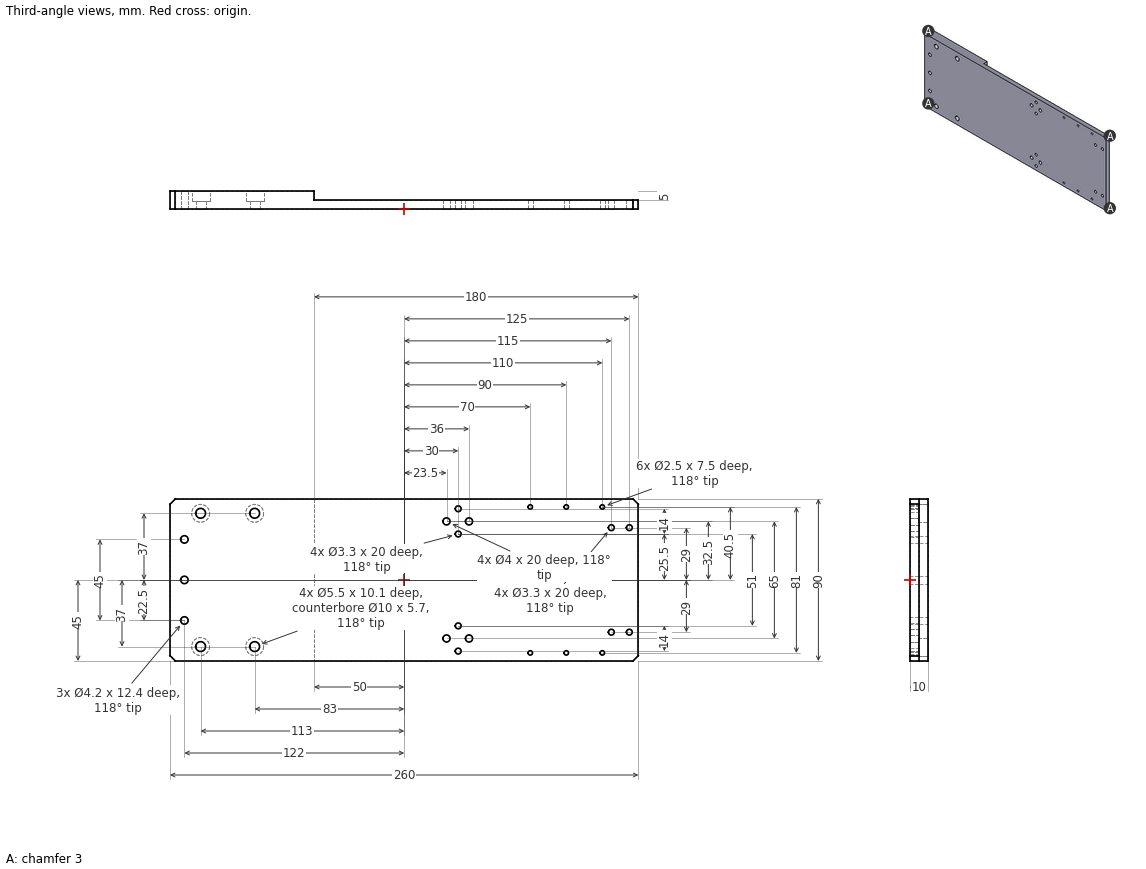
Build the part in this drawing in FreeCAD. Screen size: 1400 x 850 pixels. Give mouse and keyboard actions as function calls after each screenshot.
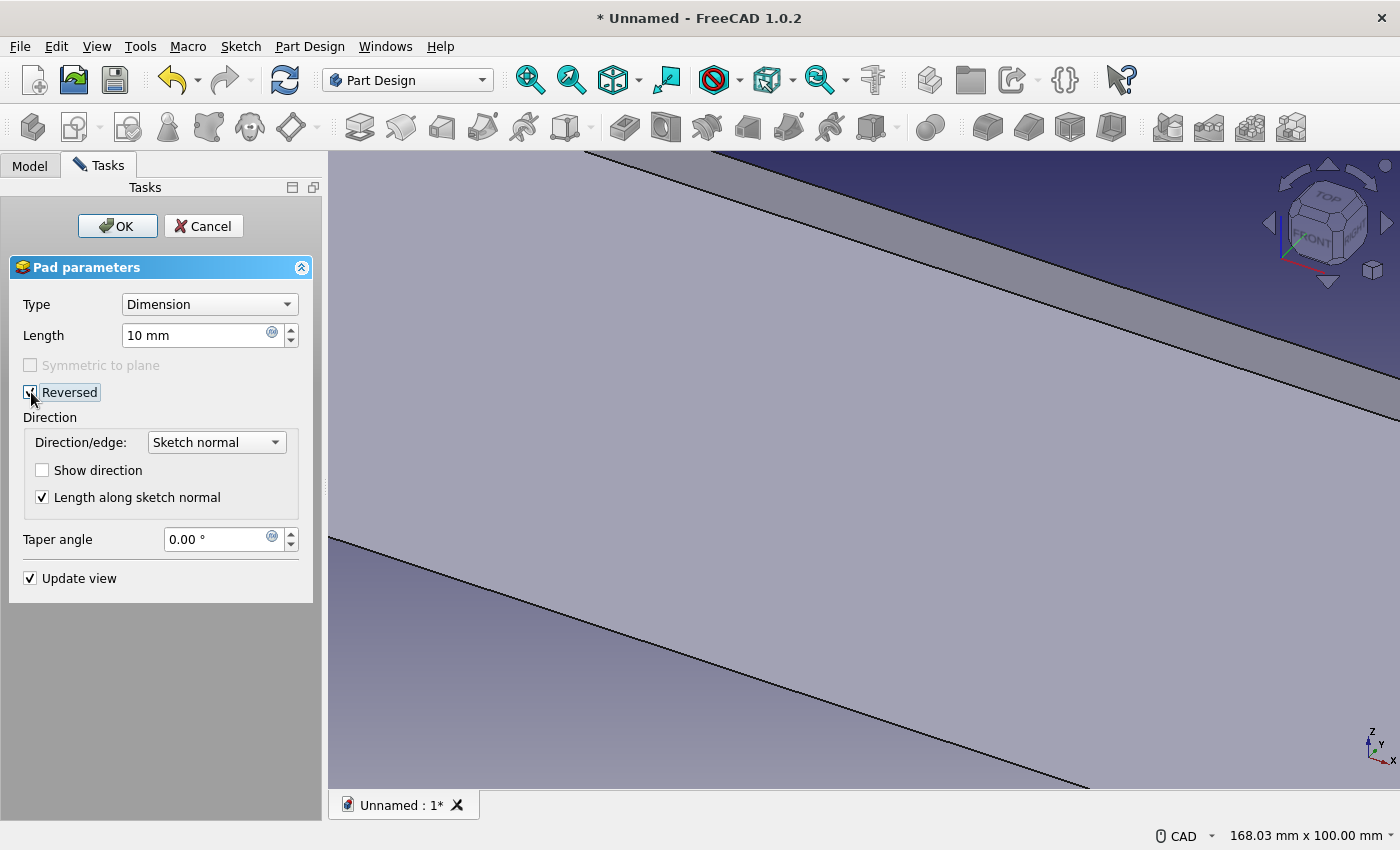
click(118, 226)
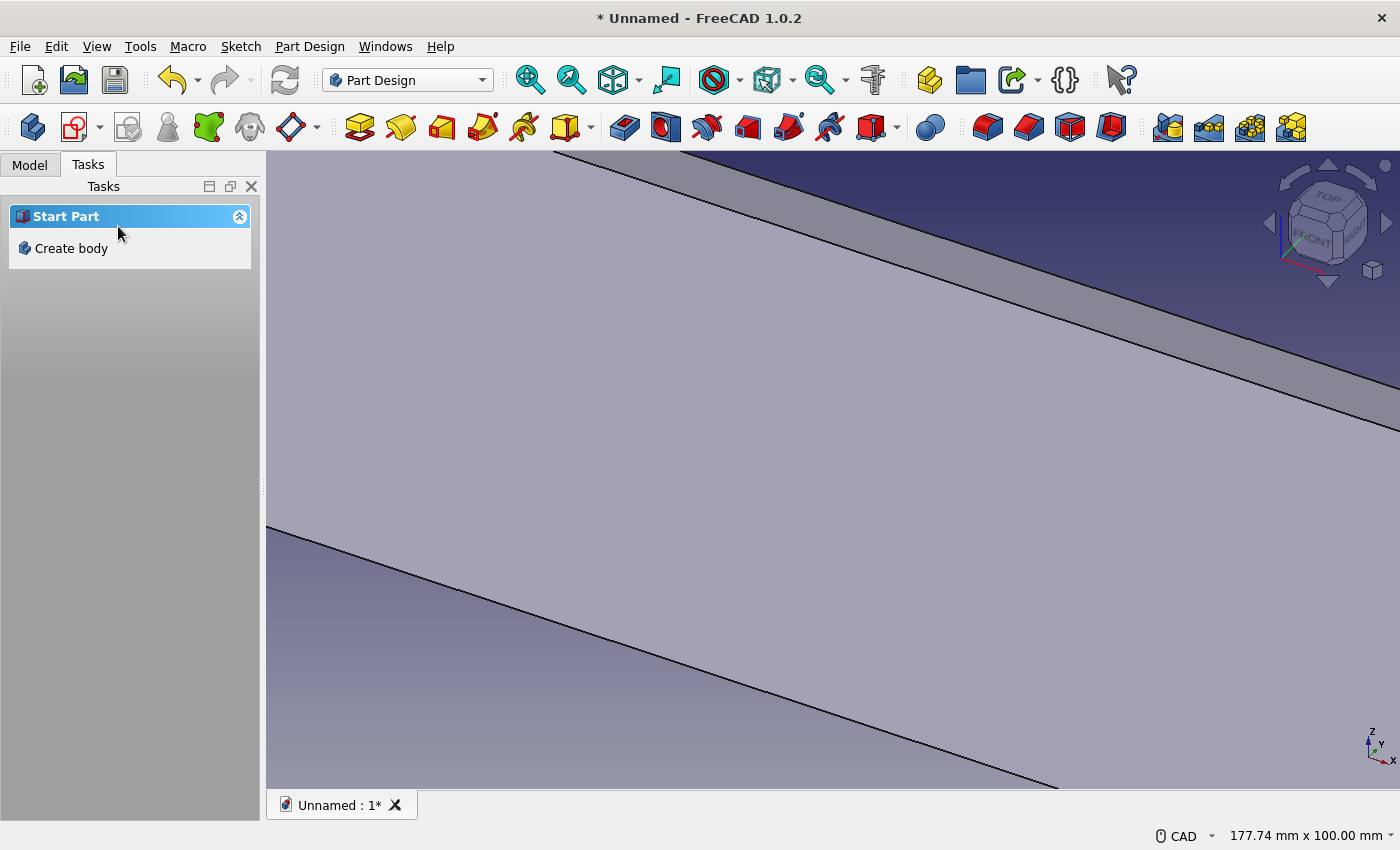
click(531, 80)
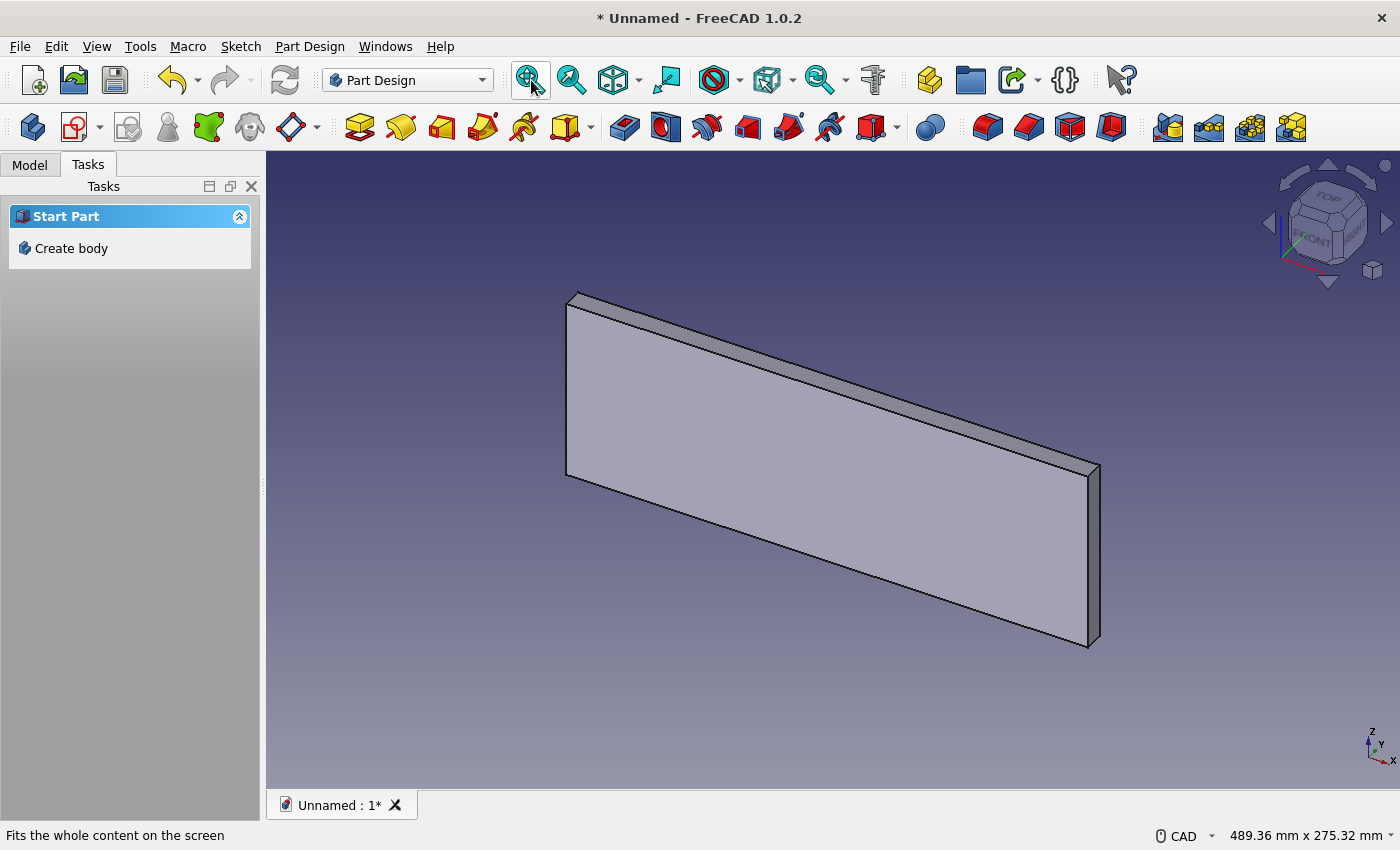
click(1094, 470)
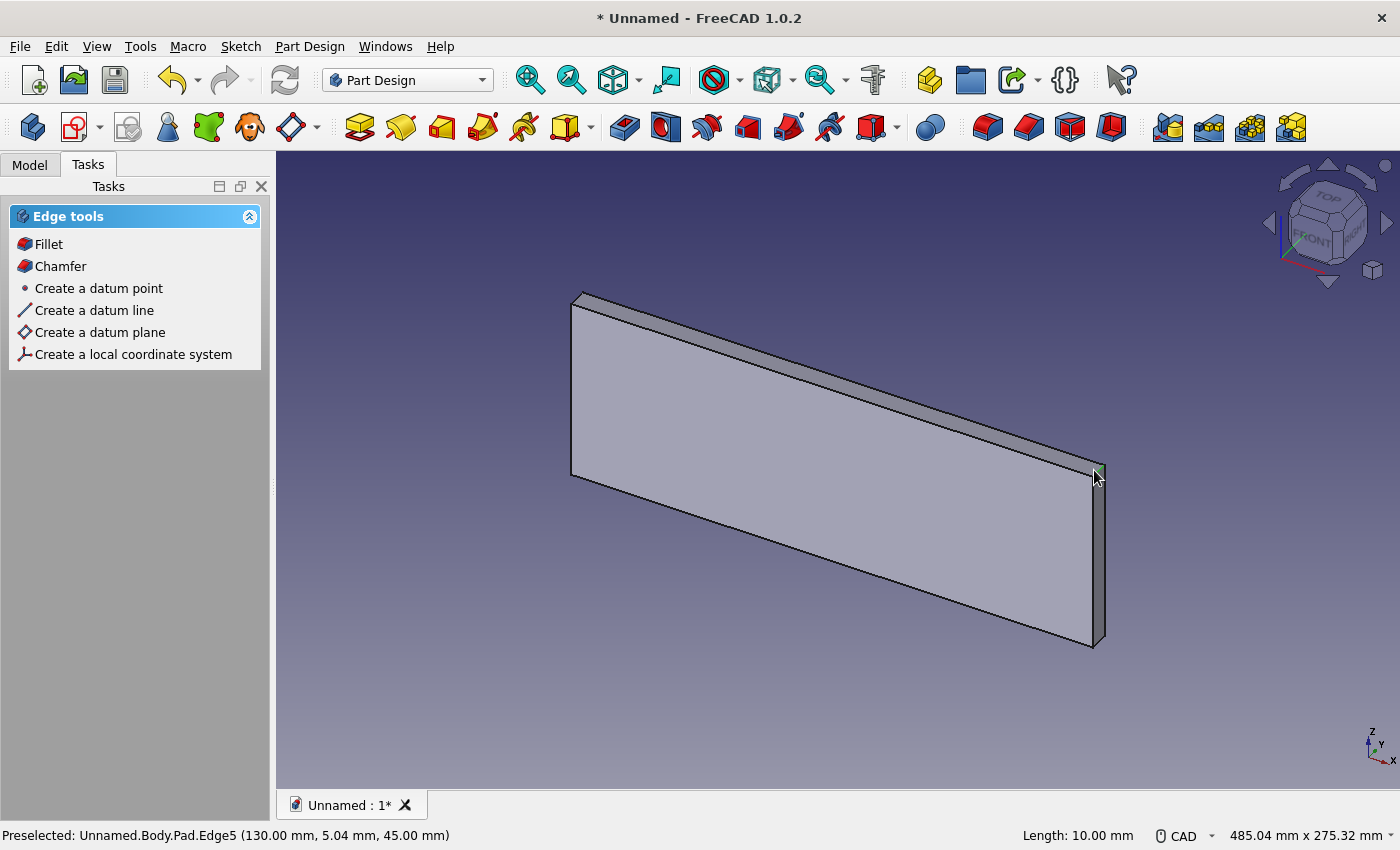
key(0)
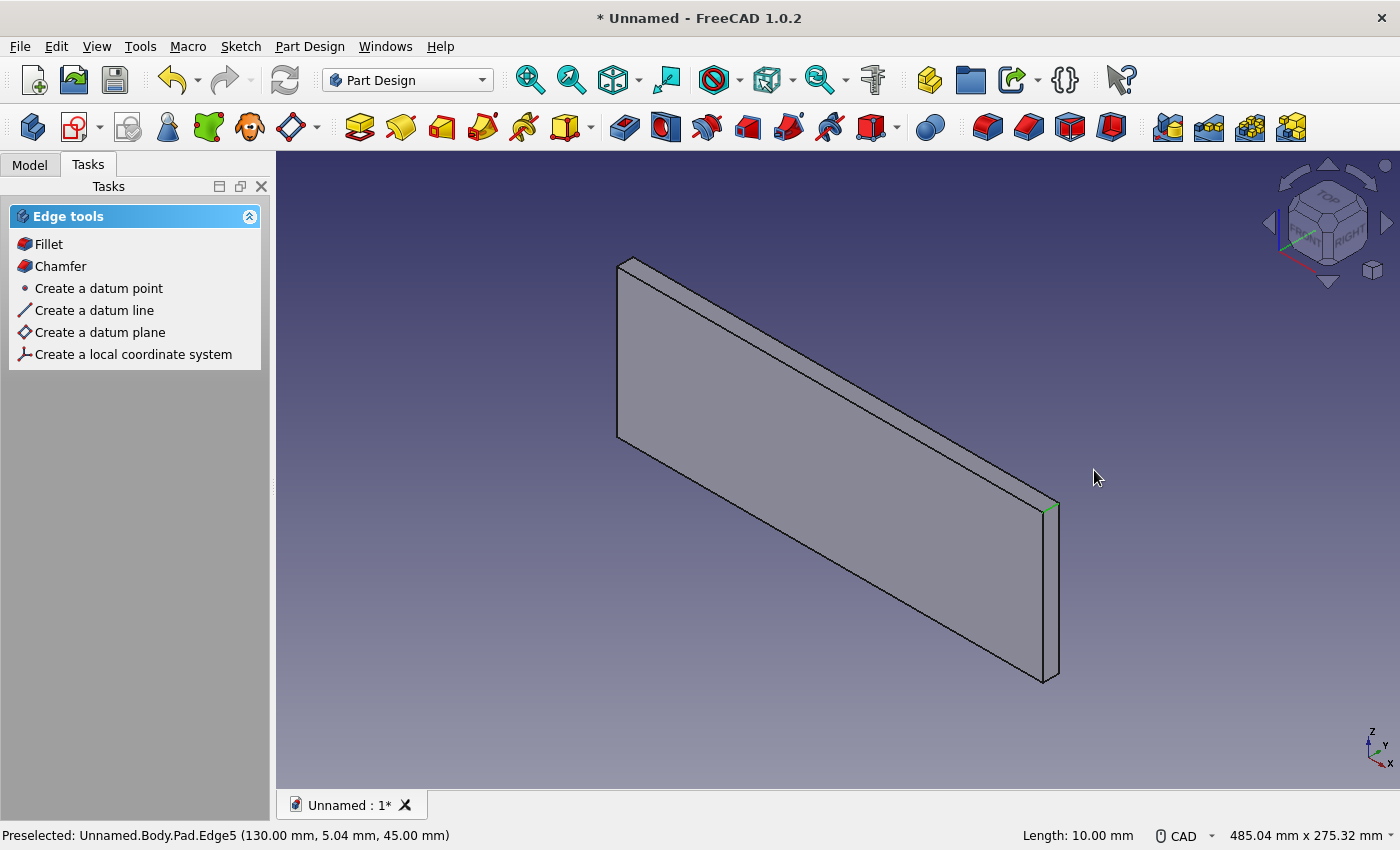
key(2)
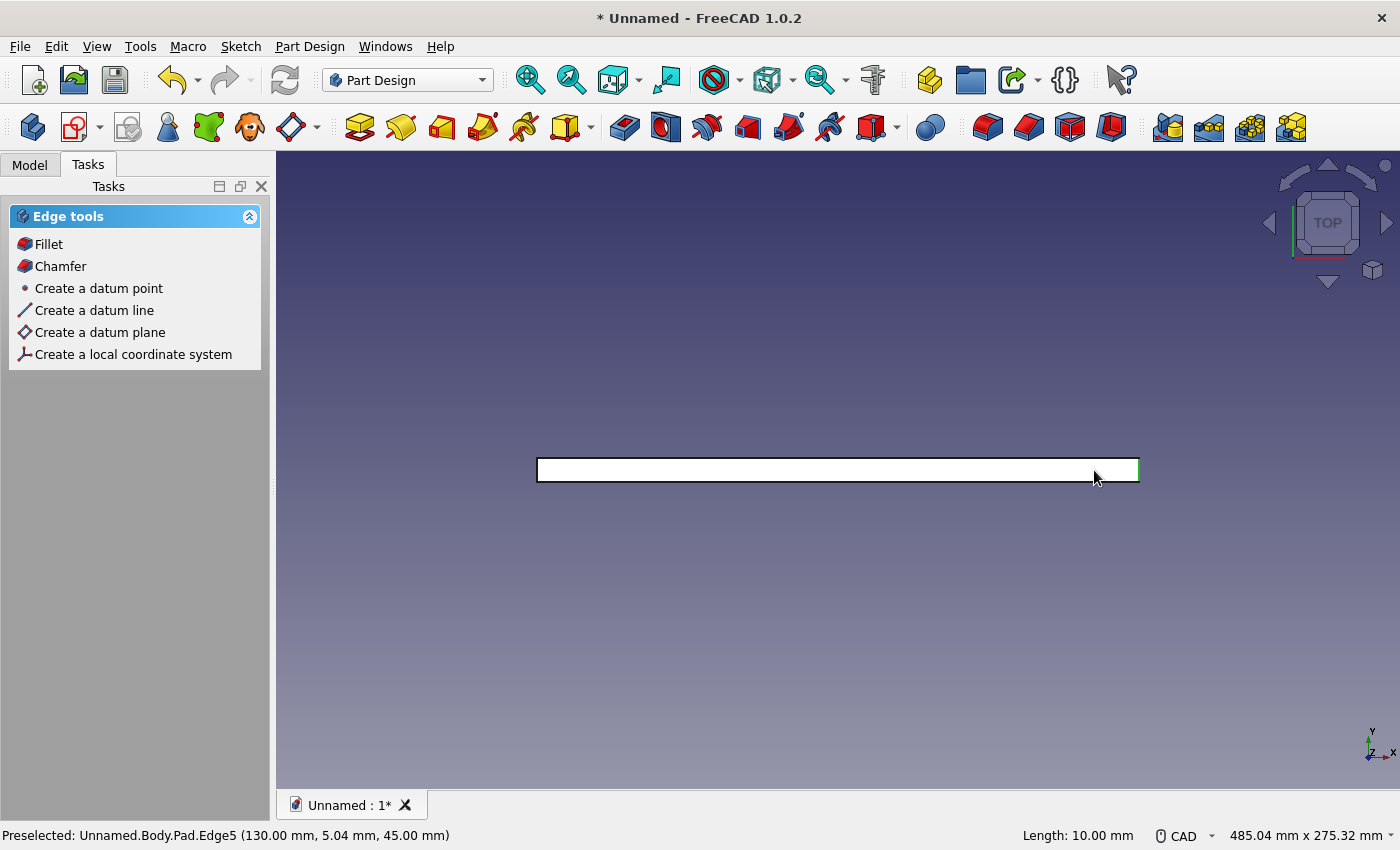
click(537, 469, ctrl)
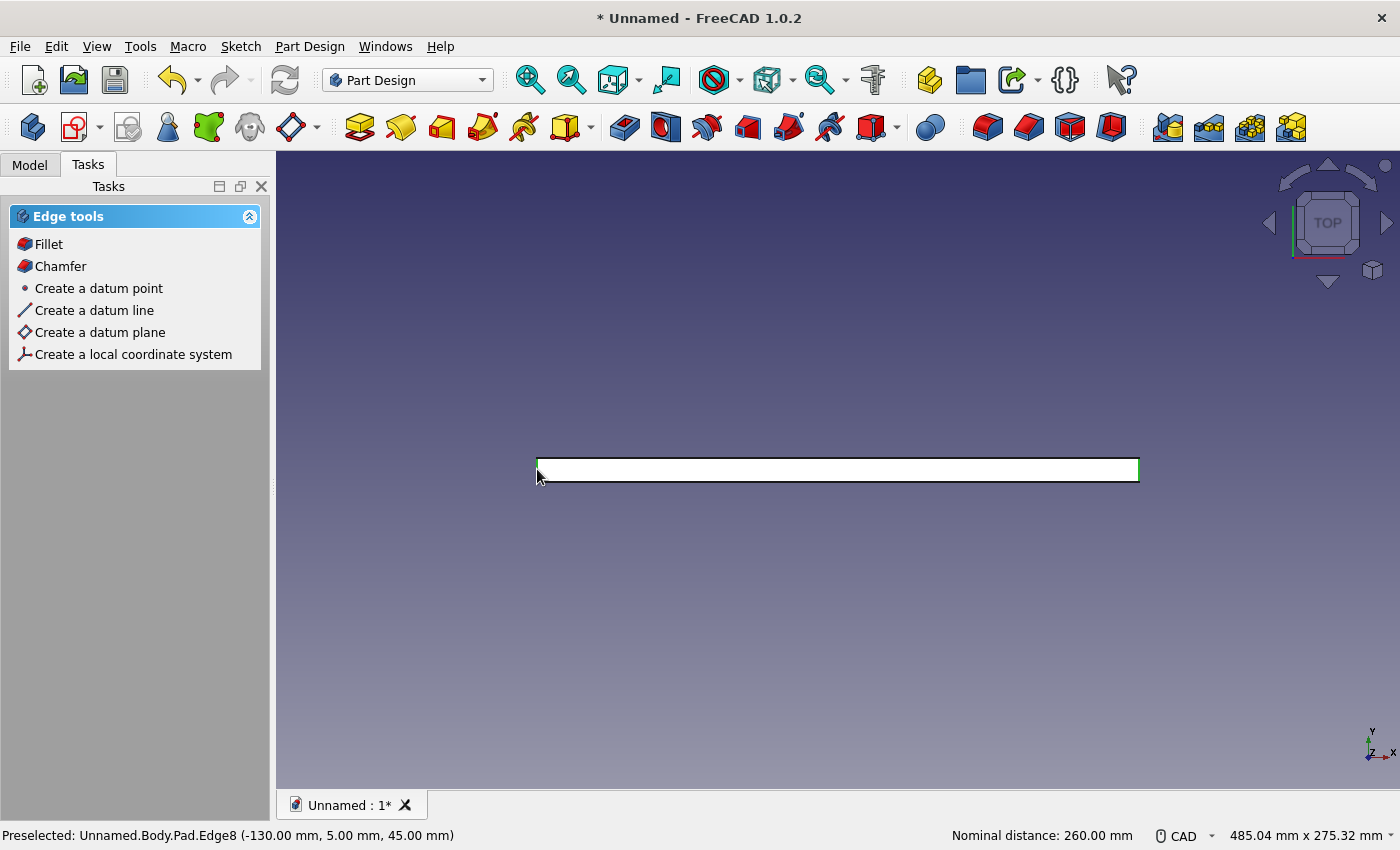
key(1)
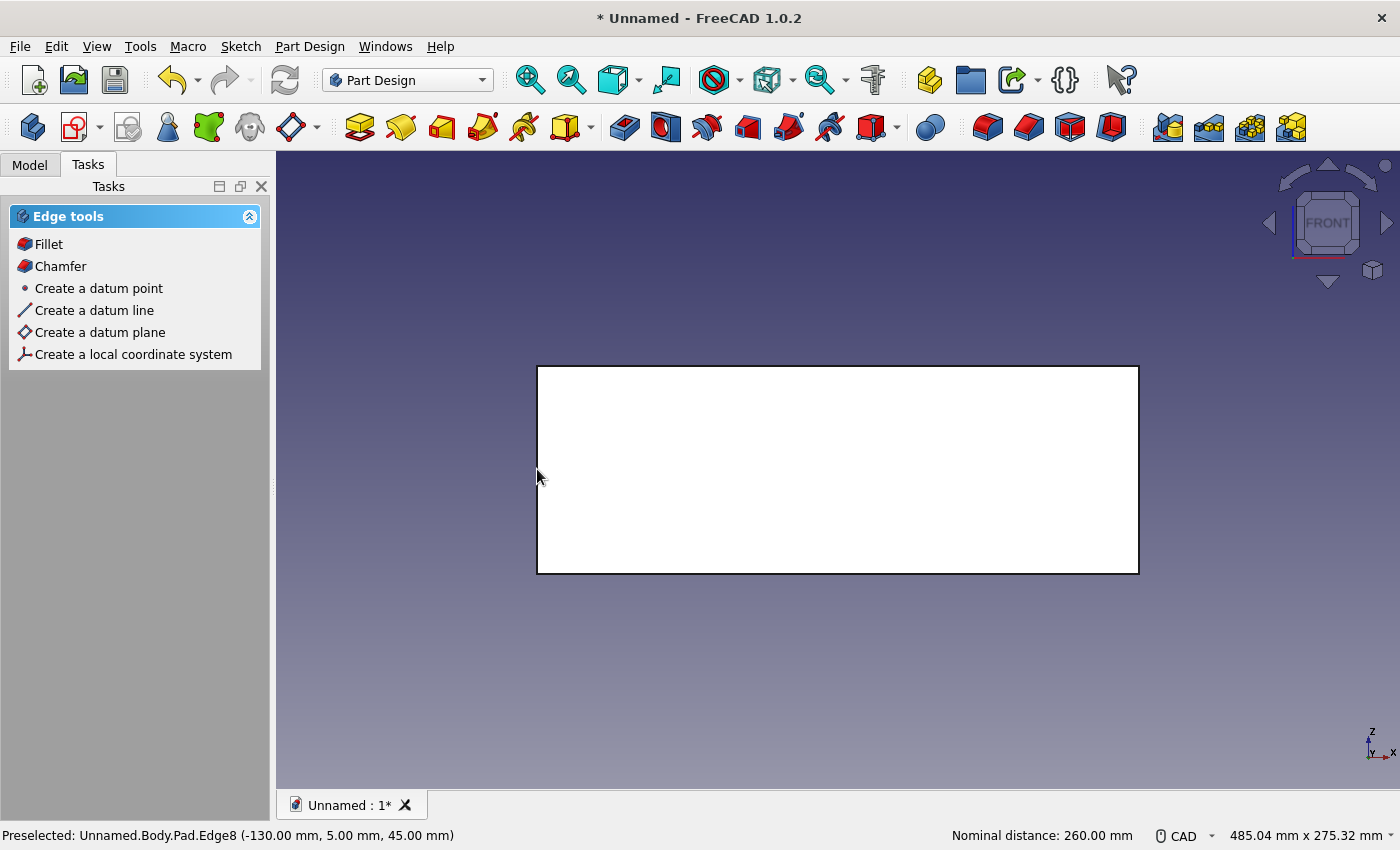
key(3)